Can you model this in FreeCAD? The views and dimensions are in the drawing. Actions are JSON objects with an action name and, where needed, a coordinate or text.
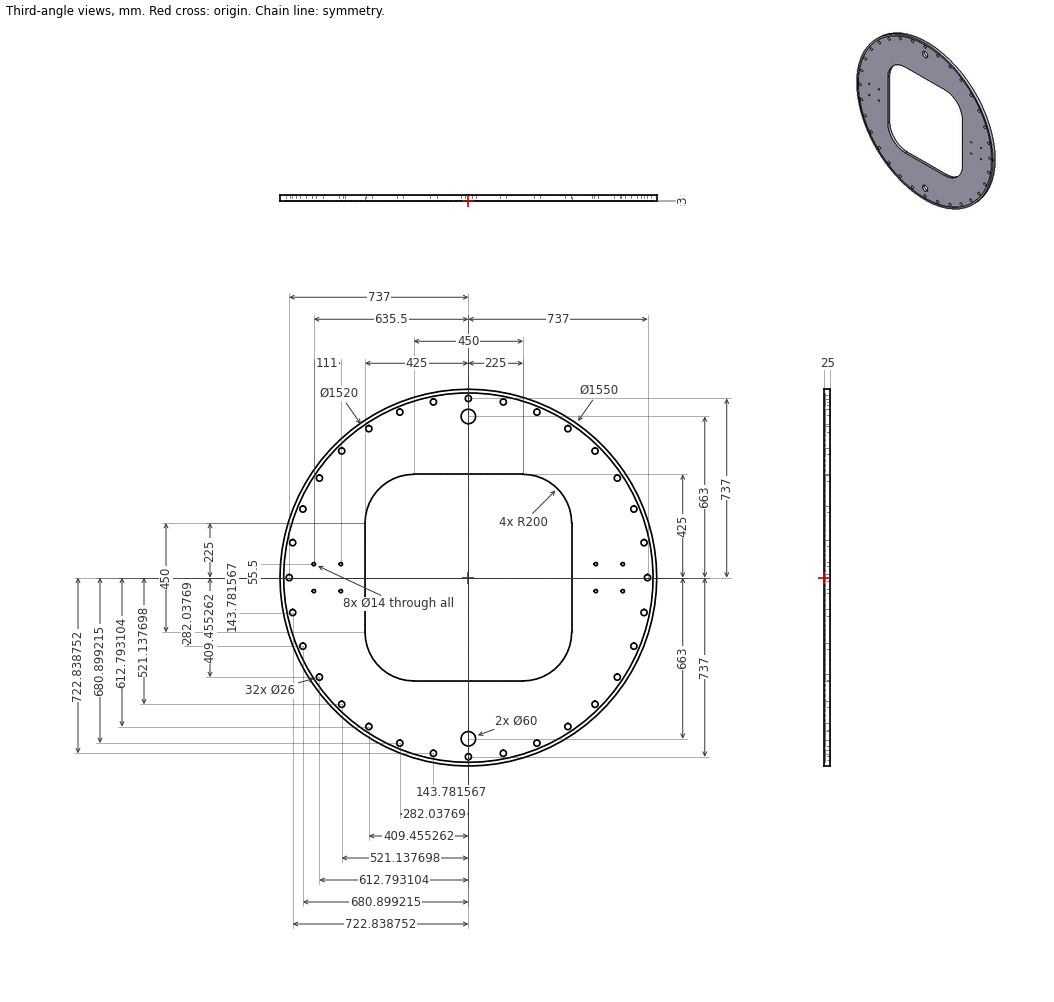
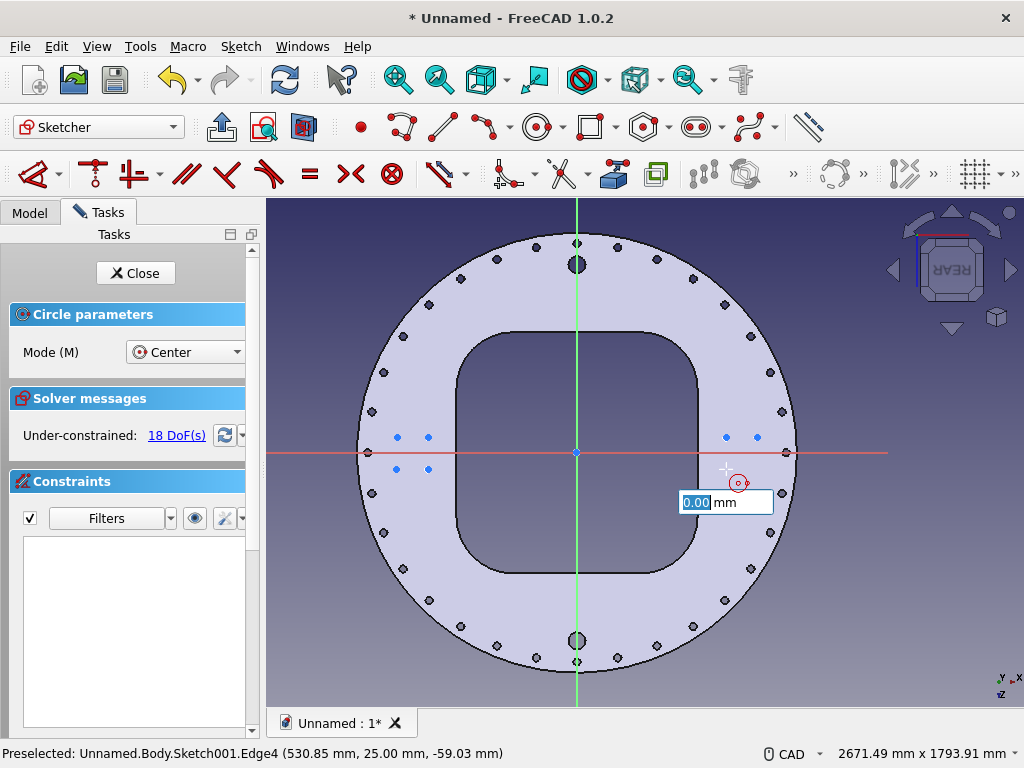
{"action": "scroll", "coordinate": [727, 467], "scroll_direction": "up", "scroll_amount": 11}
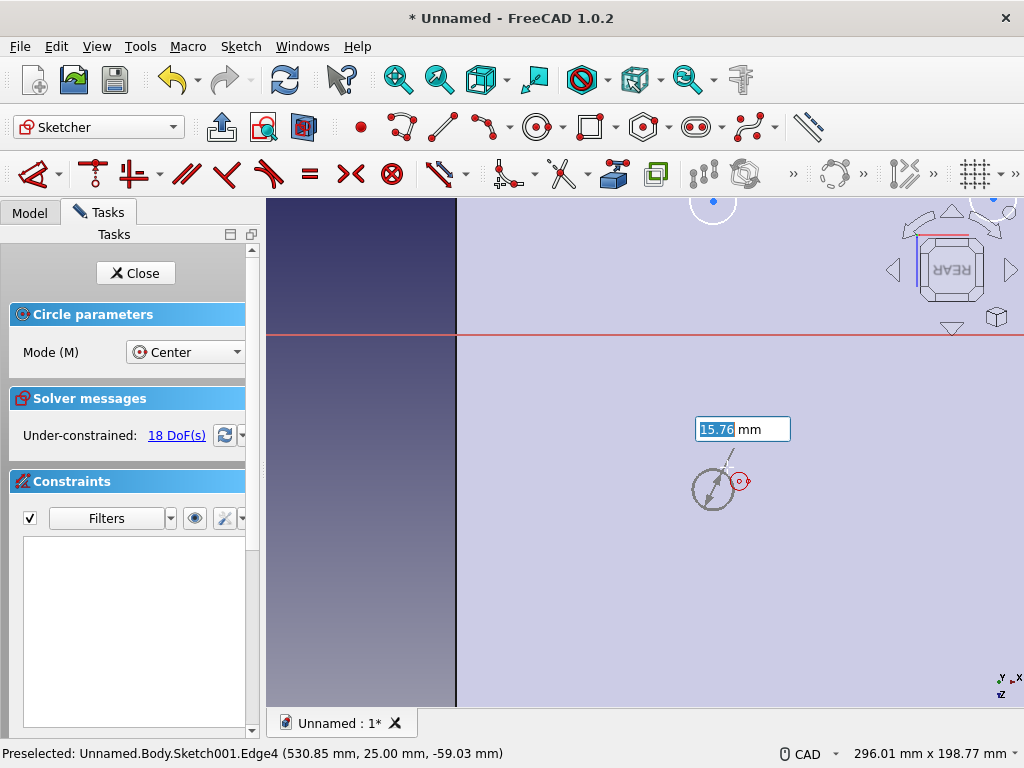
{"action": "left_click", "coordinate": [724, 464]}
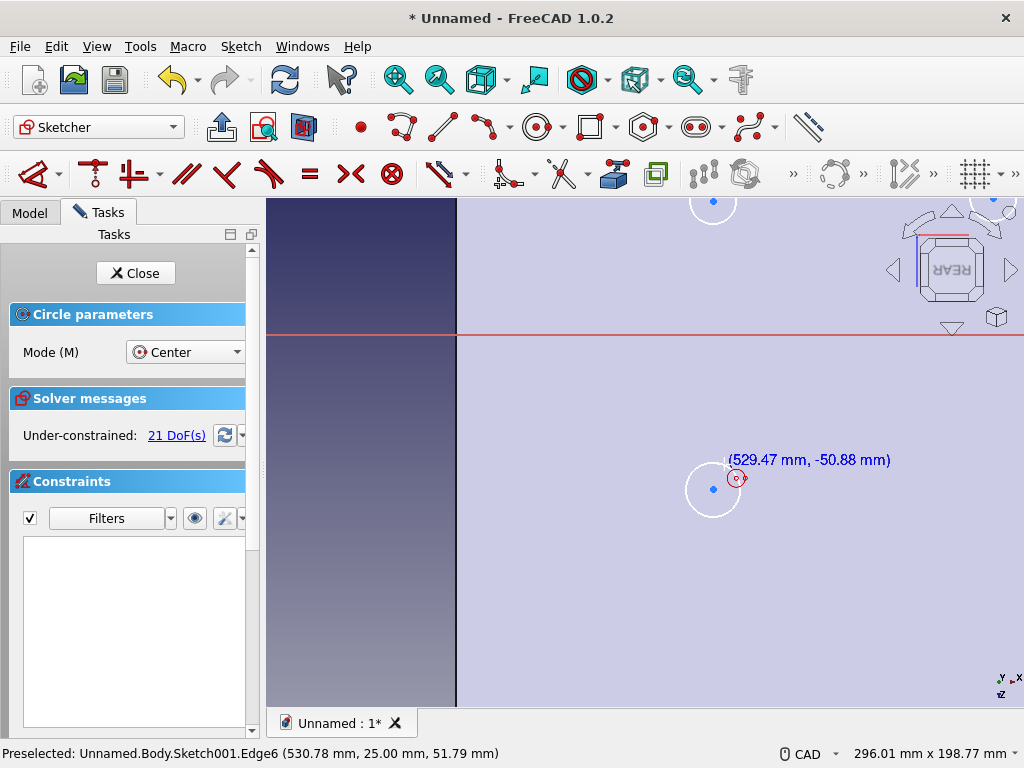
{"action": "scroll", "coordinate": [727, 467], "scroll_direction": "down", "scroll_amount": 11}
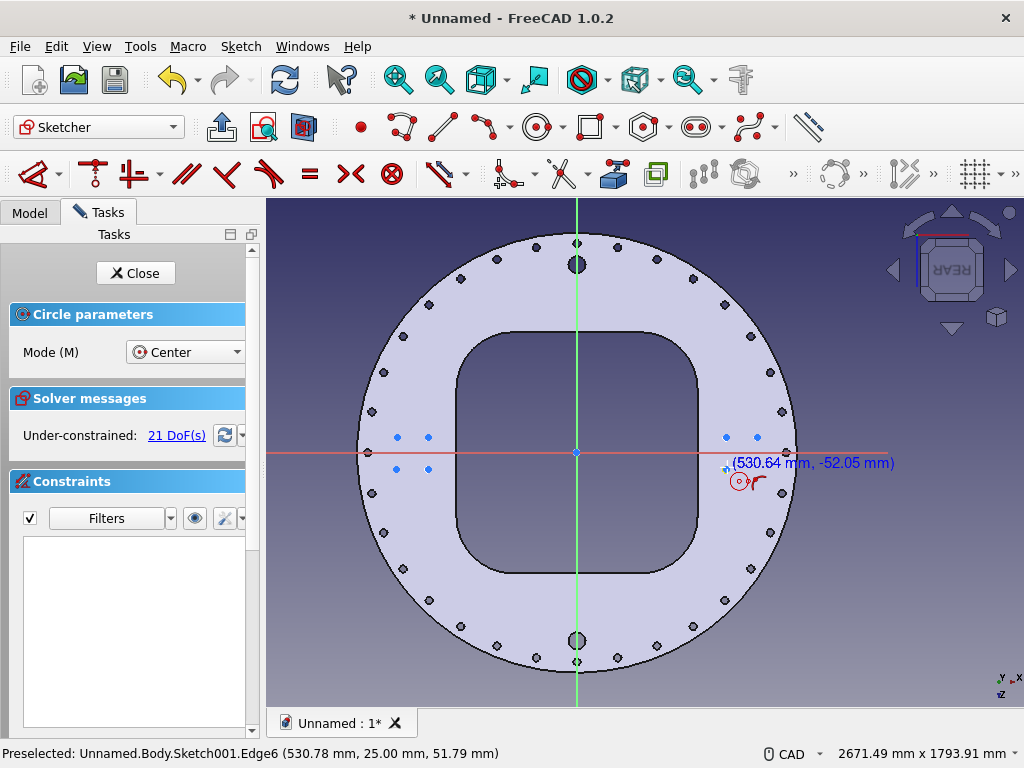
{"action": "scroll", "coordinate": [757, 469], "scroll_direction": "up", "scroll_amount": 13}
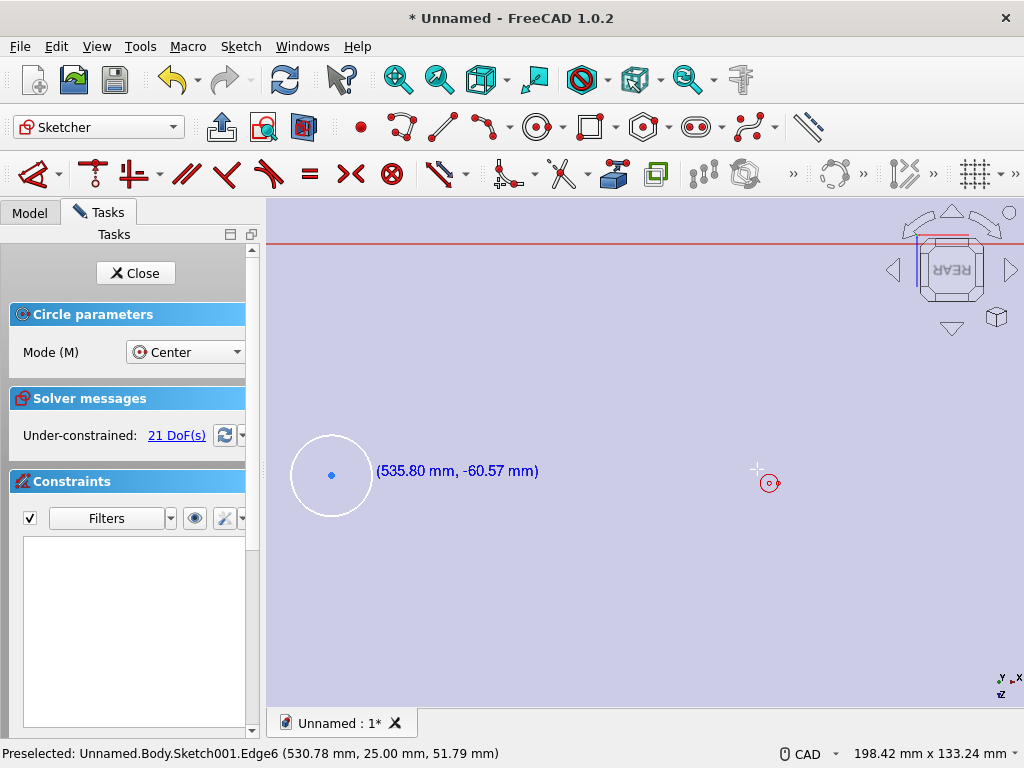
{"action": "scroll", "coordinate": [757, 469], "scroll_direction": "down", "scroll_amount": 13}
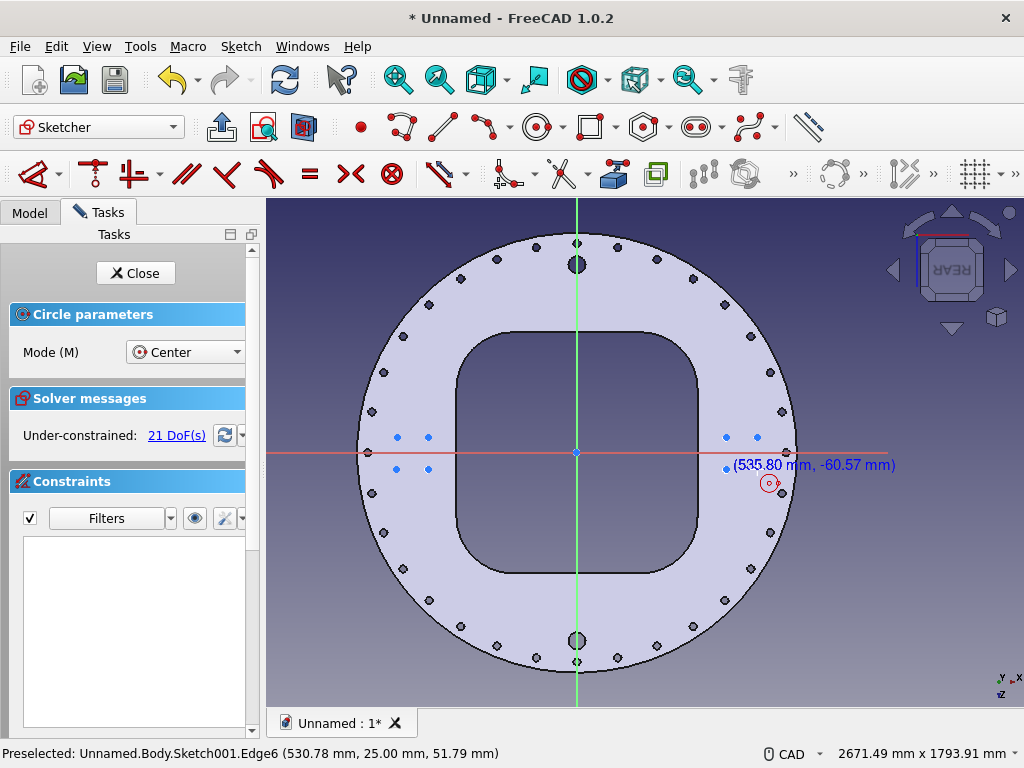
{"action": "left_click", "coordinate": [757, 469]}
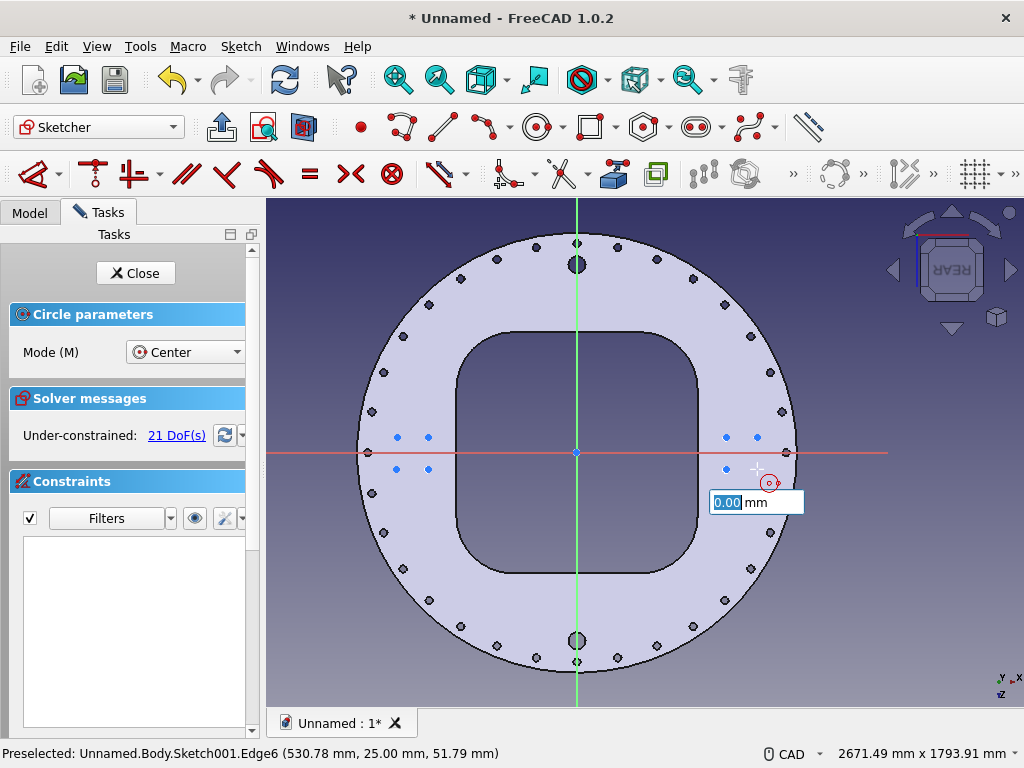
{"action": "scroll", "coordinate": [759, 467], "scroll_direction": "up", "scroll_amount": 11}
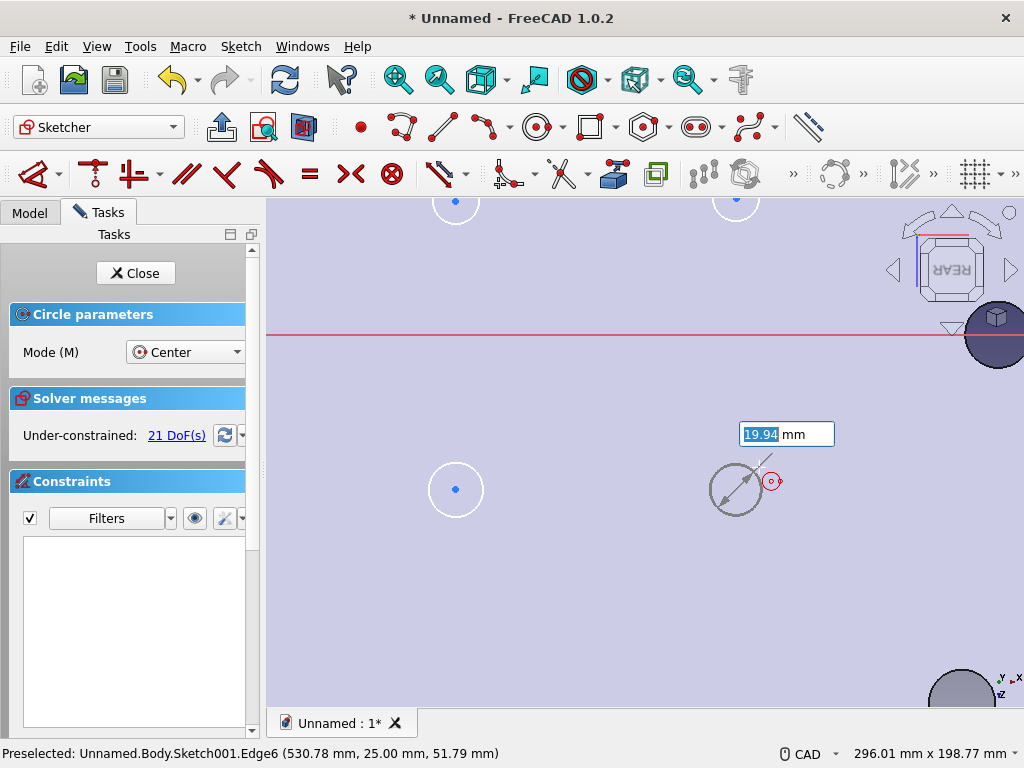
{"action": "left_click", "coordinate": [751, 464]}
{"action": "key", "text": "Escape"}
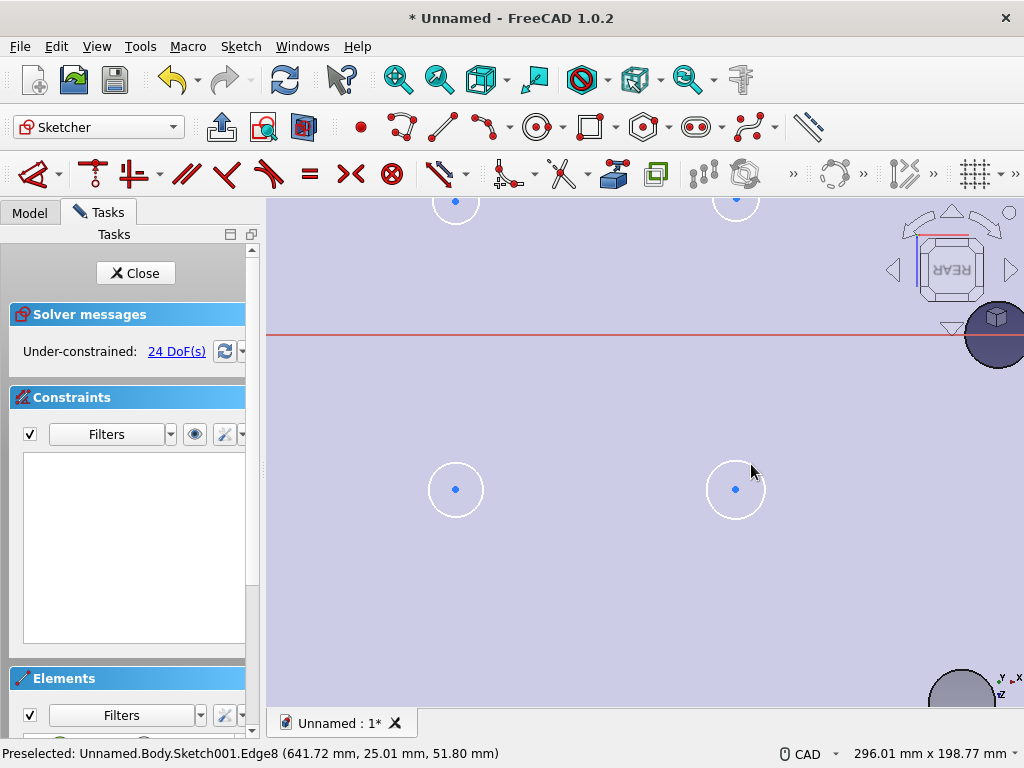
{"action": "scroll", "coordinate": [759, 467], "scroll_direction": "down", "scroll_amount": 11}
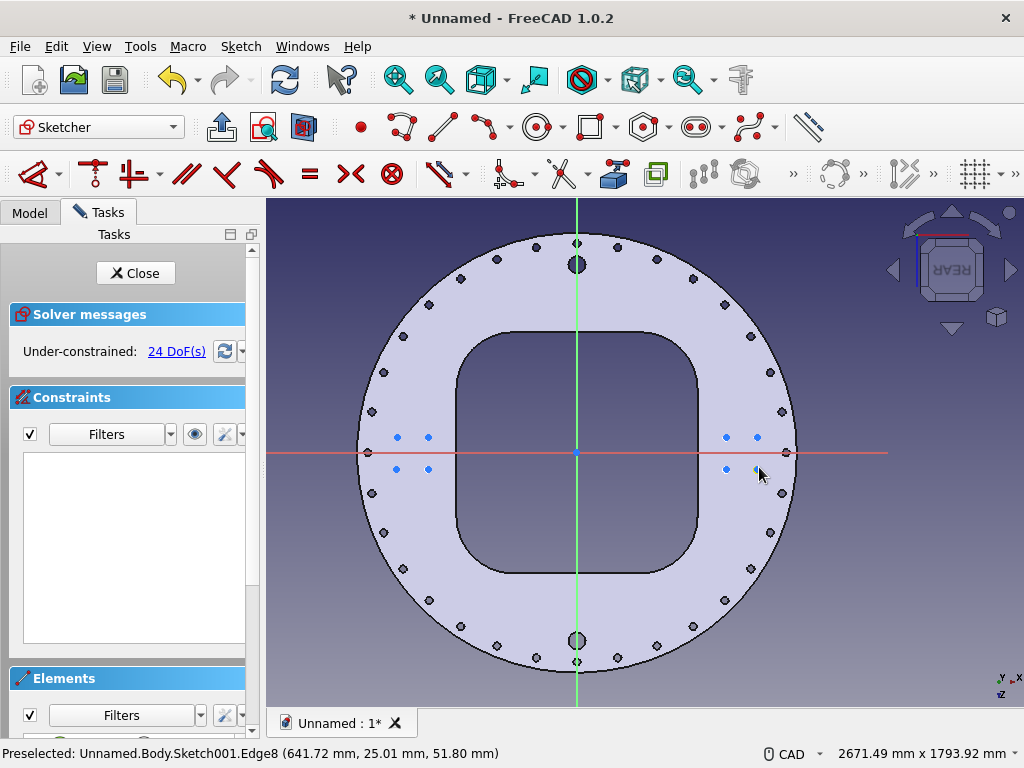
{"action": "scroll", "coordinate": [398, 468], "scroll_direction": "up", "scroll_amount": 9}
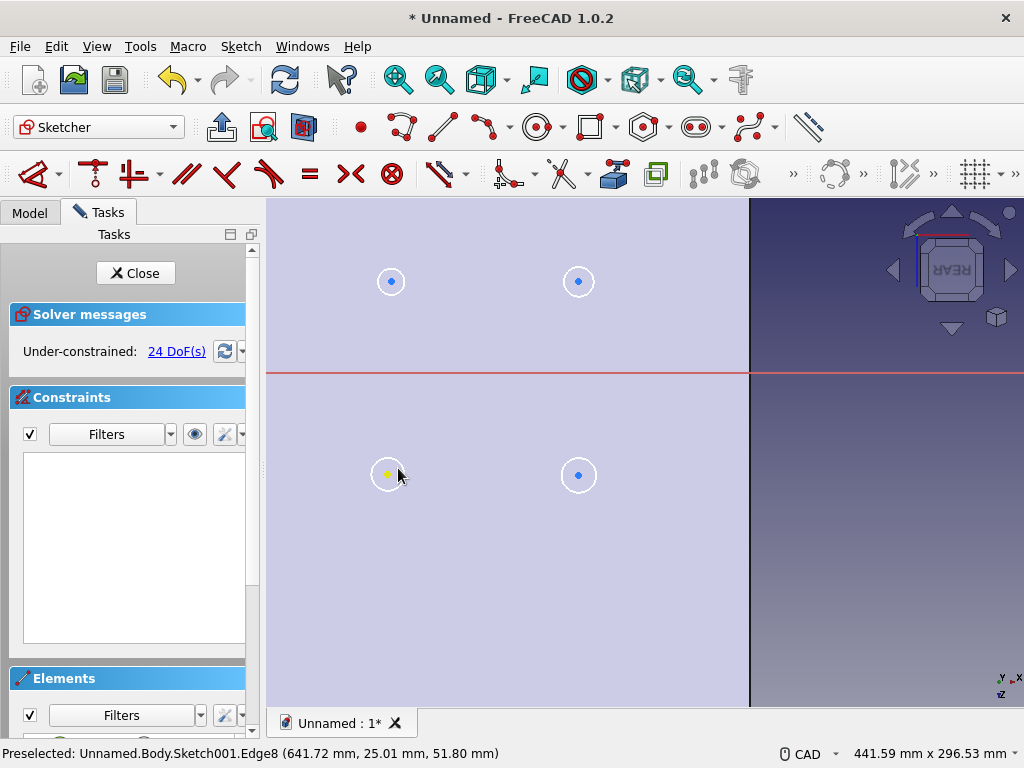
{"action": "left_click", "coordinate": [399, 463]}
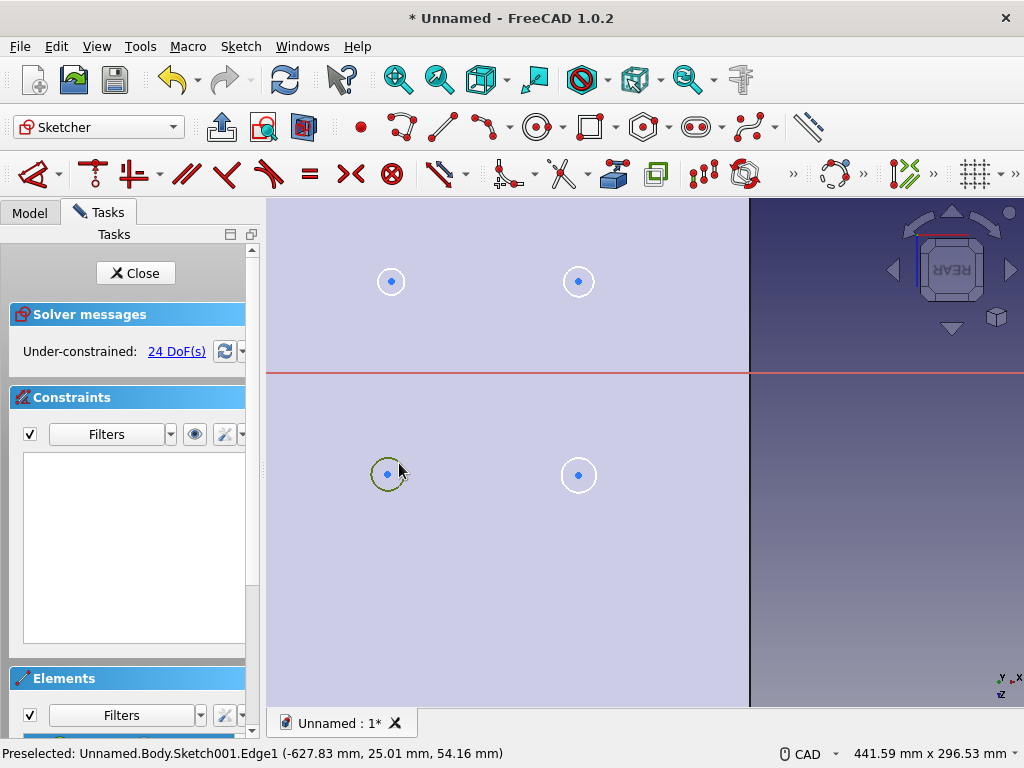
{"action": "left_click", "coordinate": [591, 463]}